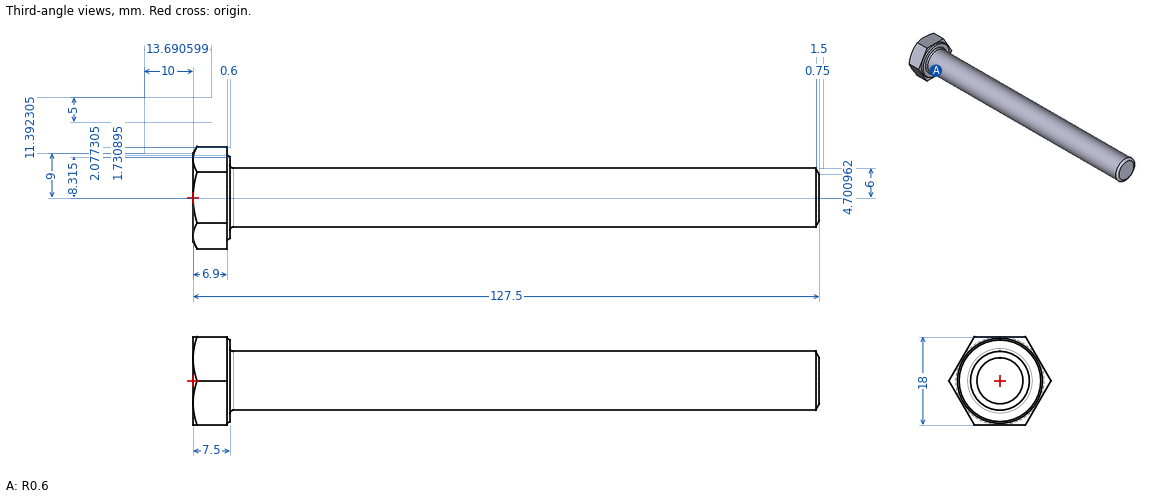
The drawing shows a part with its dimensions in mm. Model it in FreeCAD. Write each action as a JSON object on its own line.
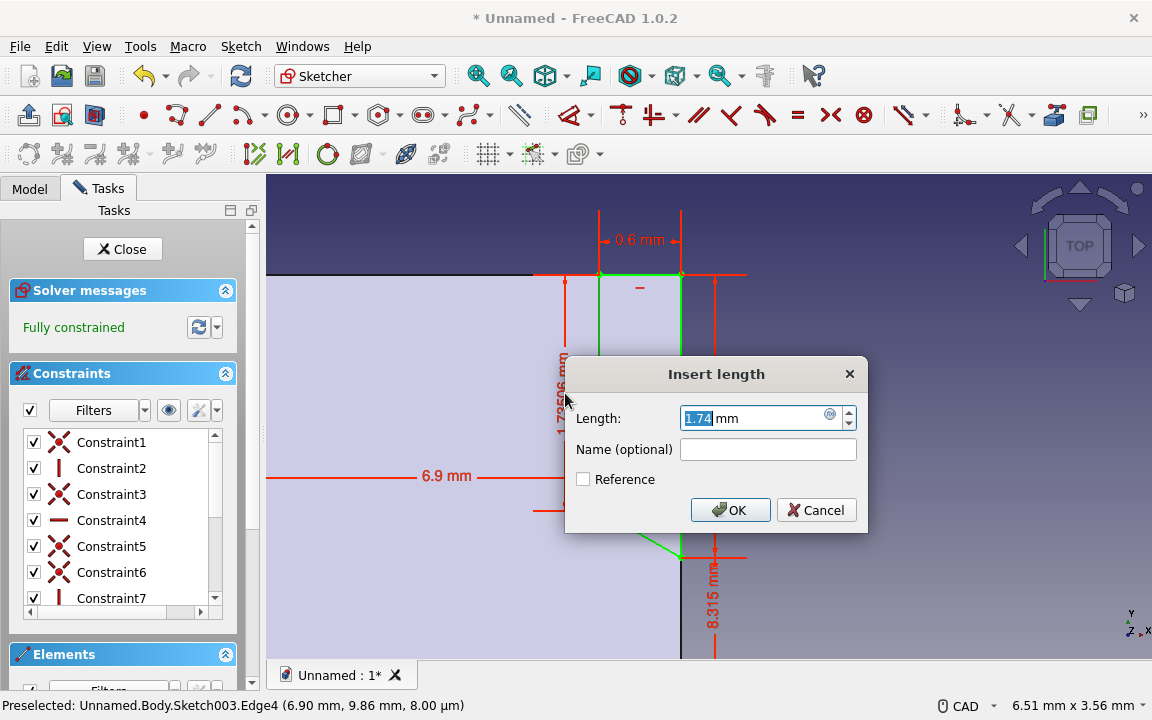
{"action": "type", "text": "1.730895"}
{"action": "key", "text": "Return"}
{"action": "key", "text": "Escape"}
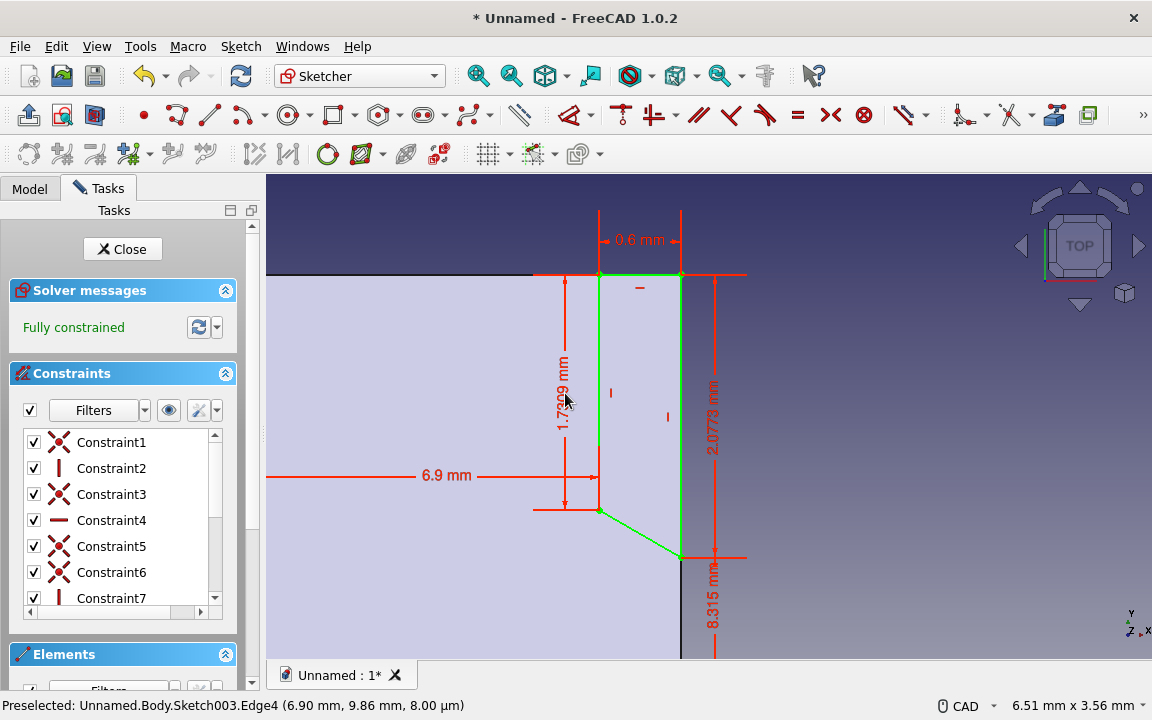
{"action": "left_click", "coordinate": [123, 249]}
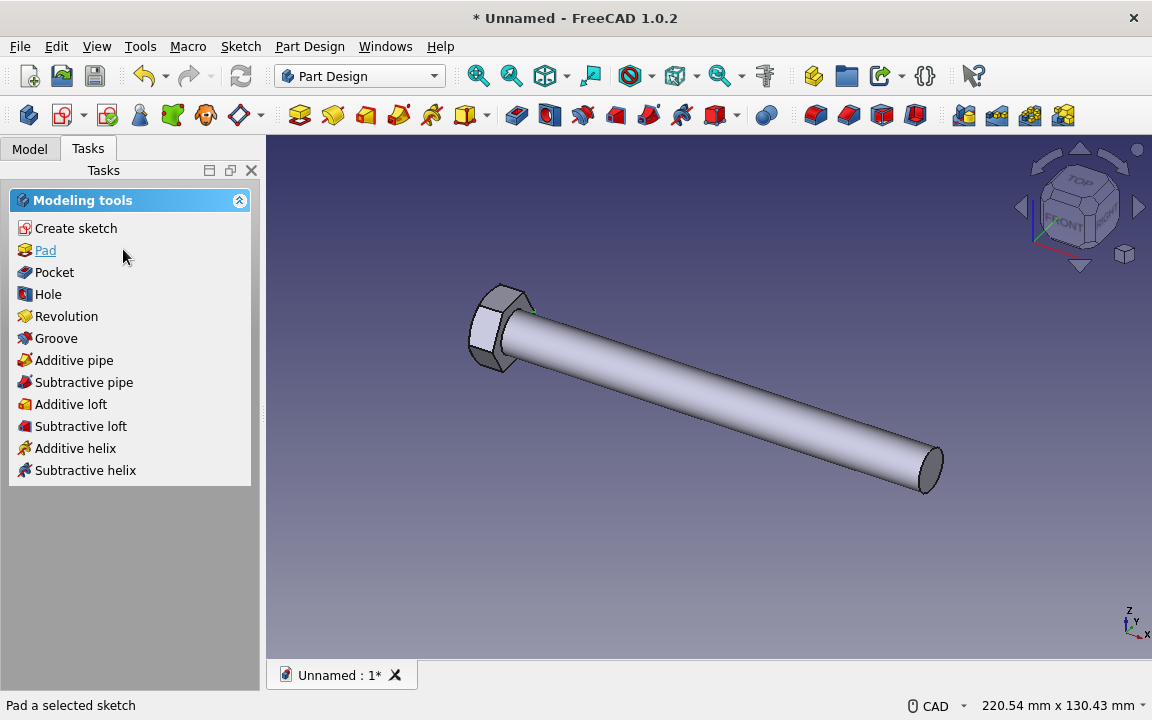
{"action": "left_click", "coordinate": [583, 116]}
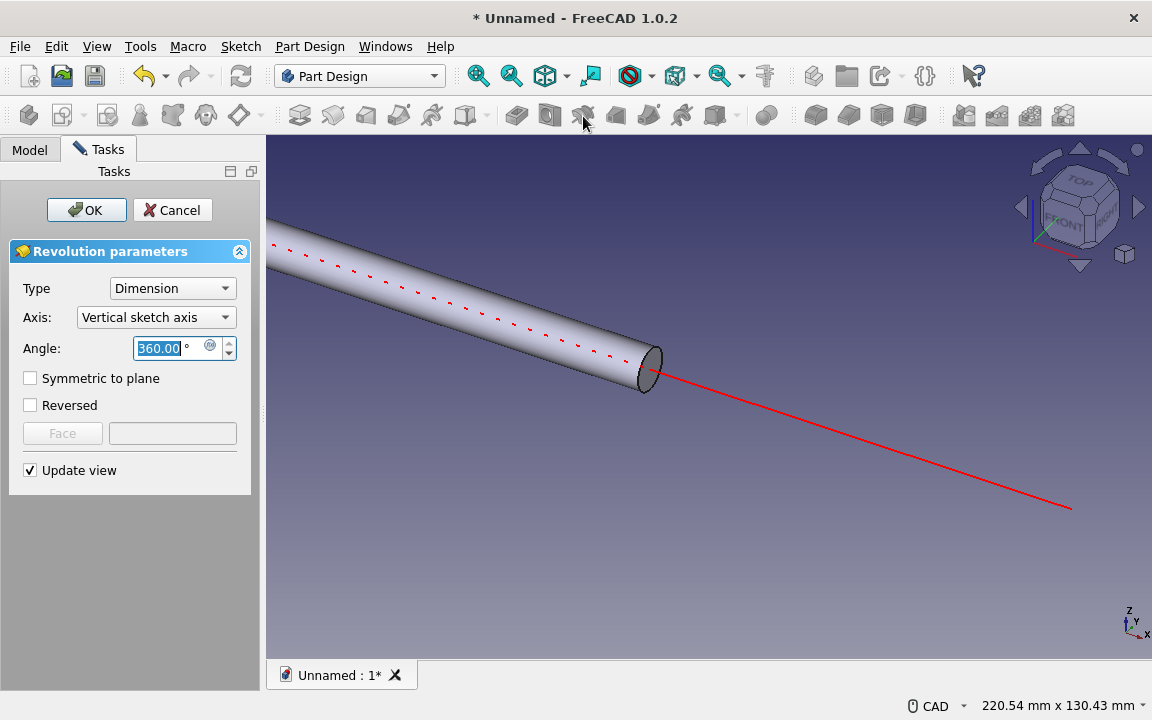
{"action": "left_click", "coordinate": [157, 318]}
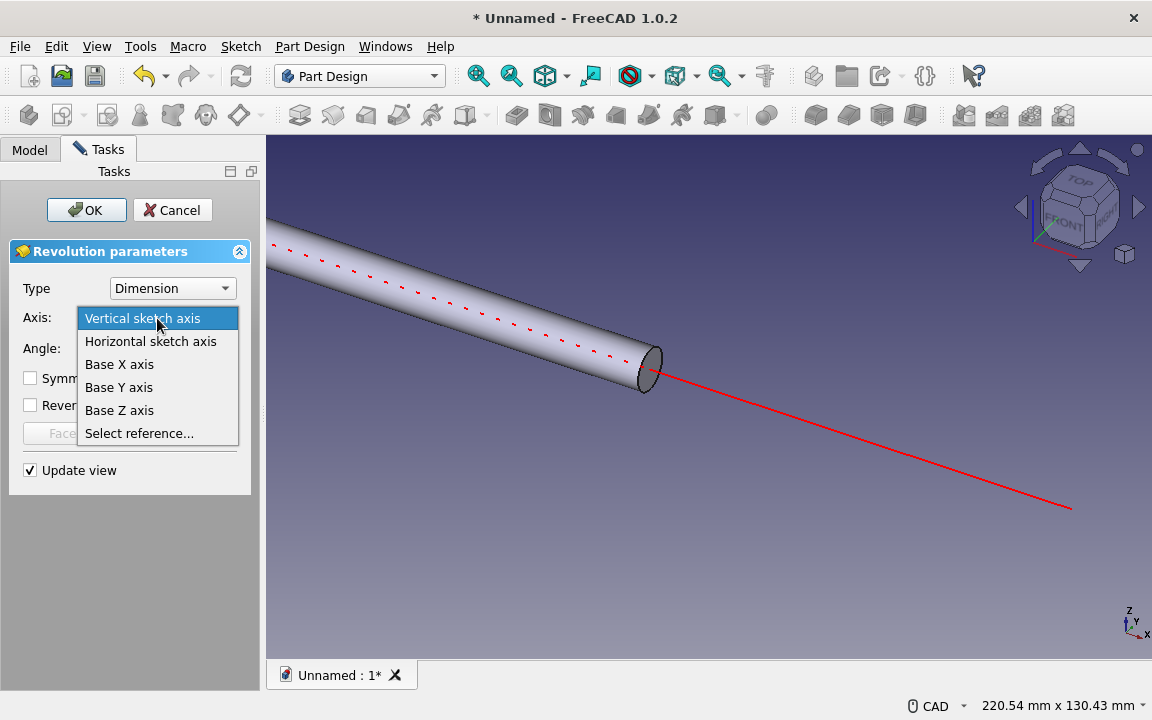
{"action": "left_click", "coordinate": [156, 342]}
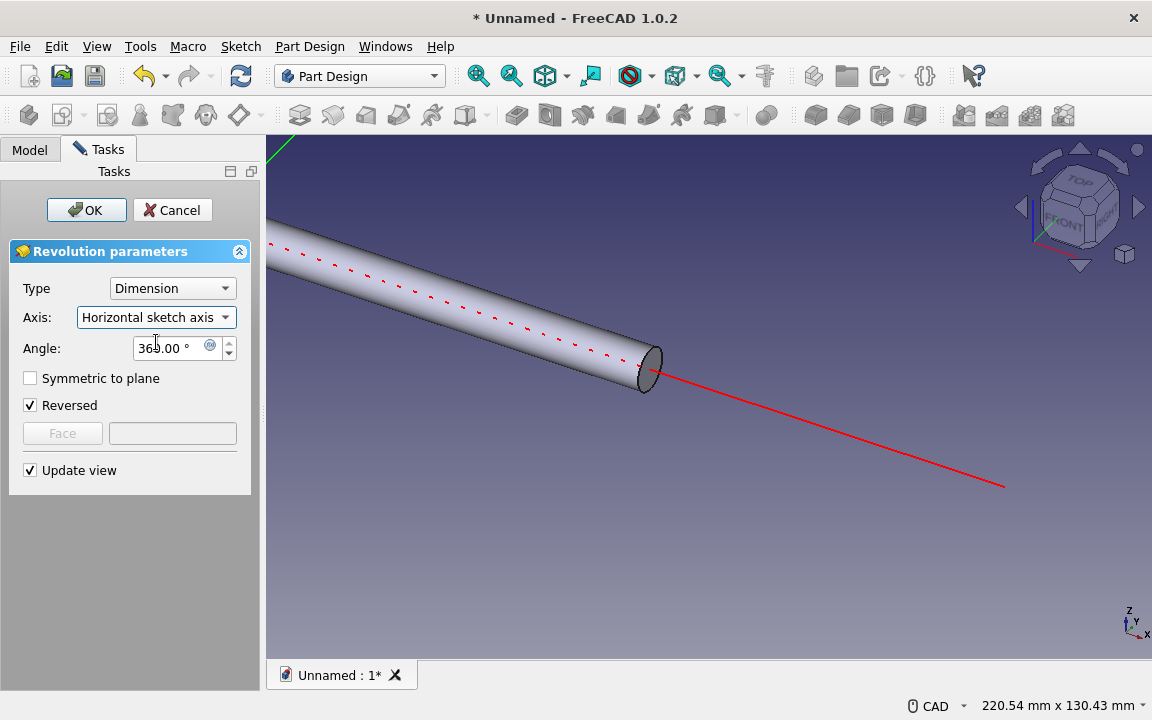
{"action": "left_click", "coordinate": [87, 210]}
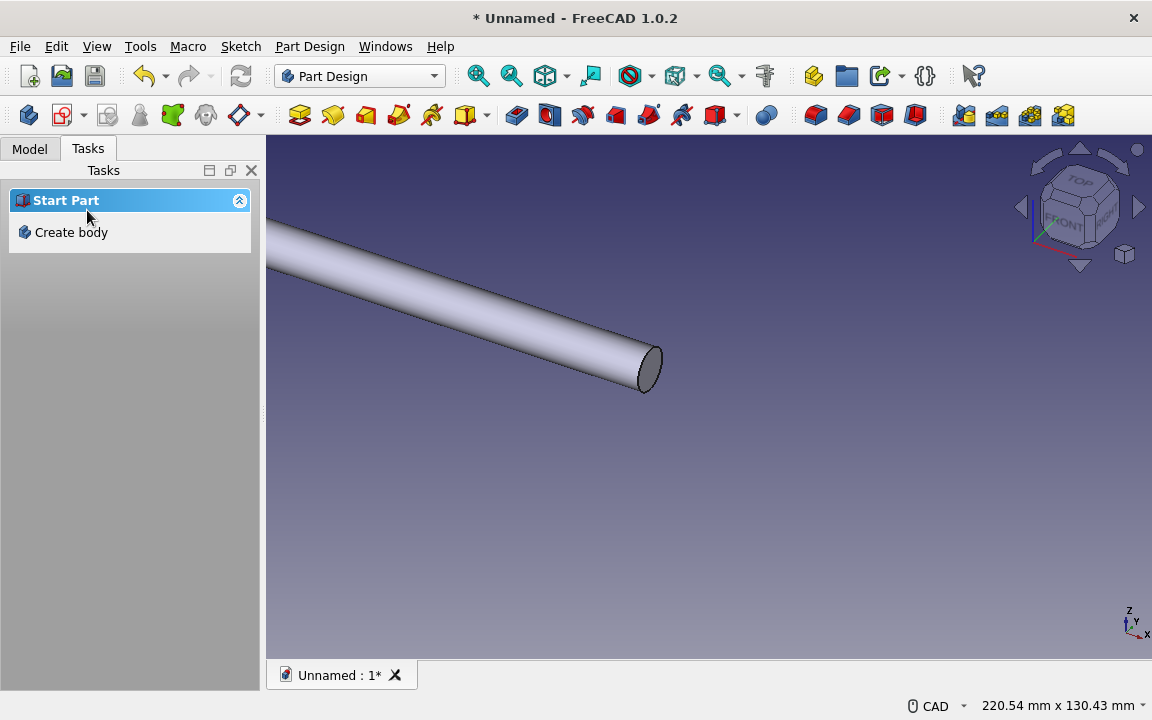
{"action": "left_click", "coordinate": [479, 76]}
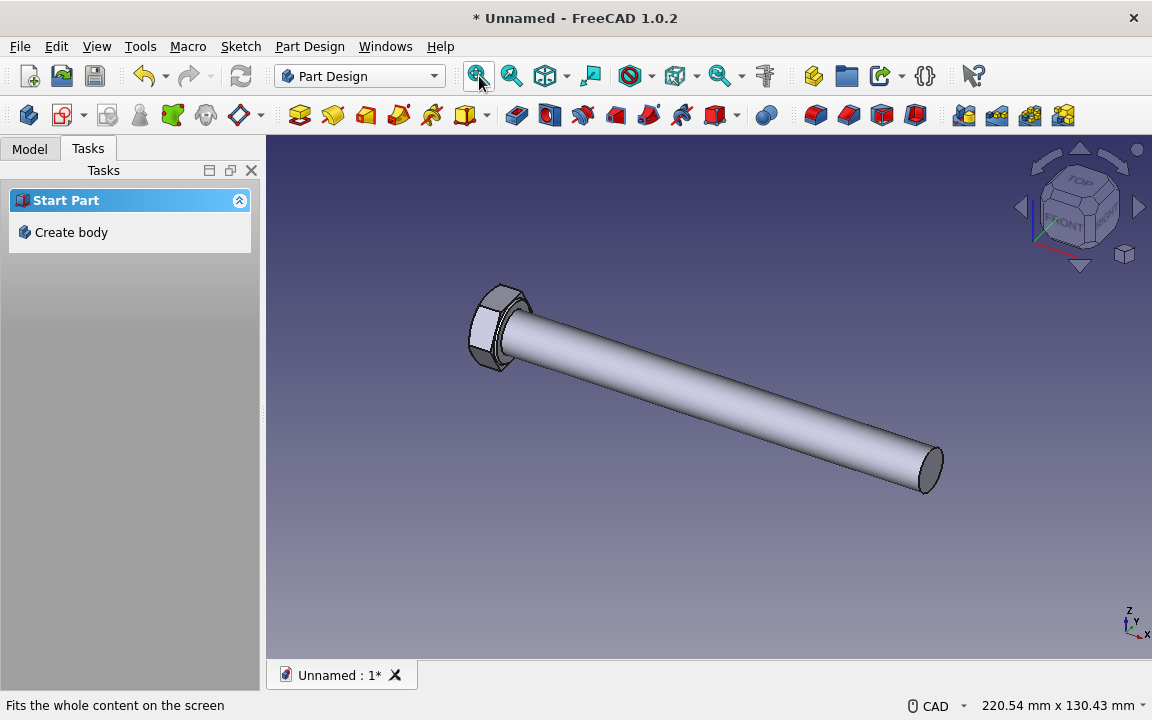
{"action": "key", "text": "0"}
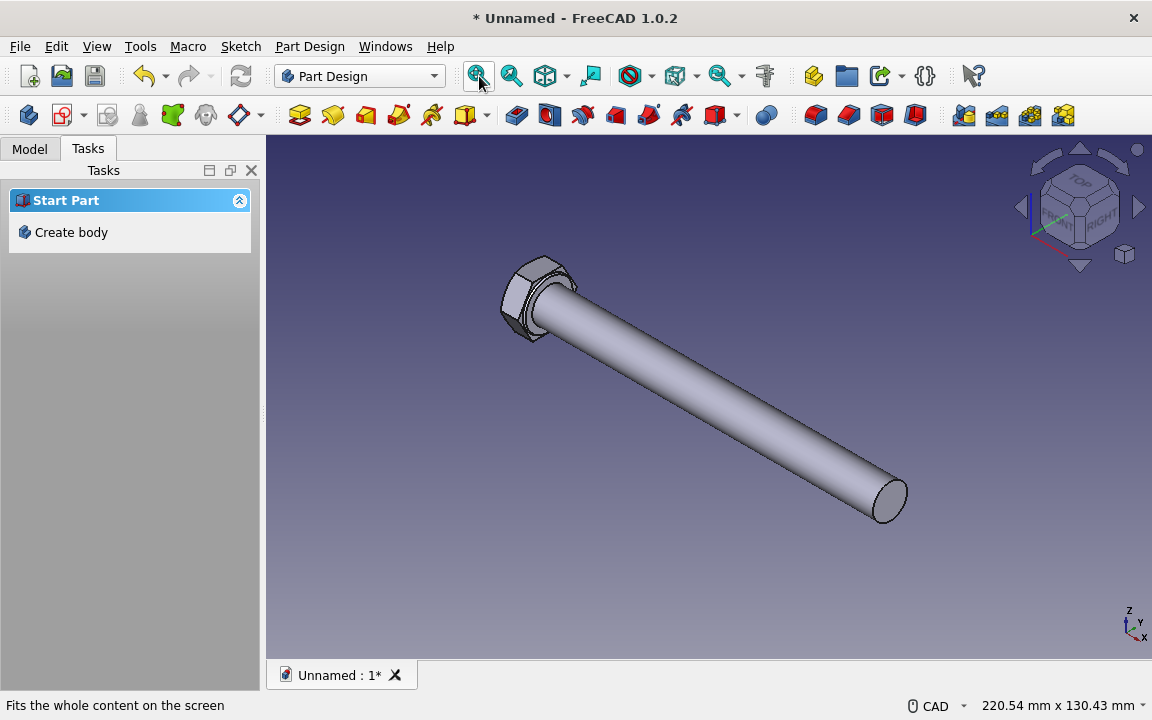
{"action": "key", "text": "2"}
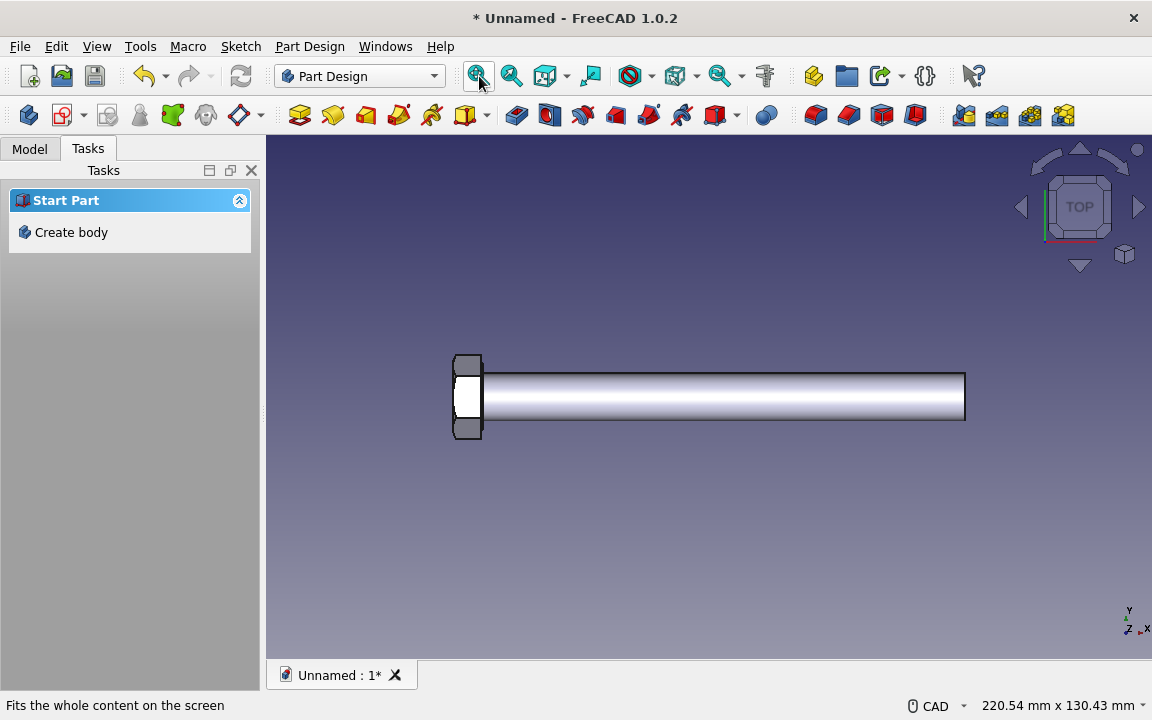
{"action": "key", "text": "1"}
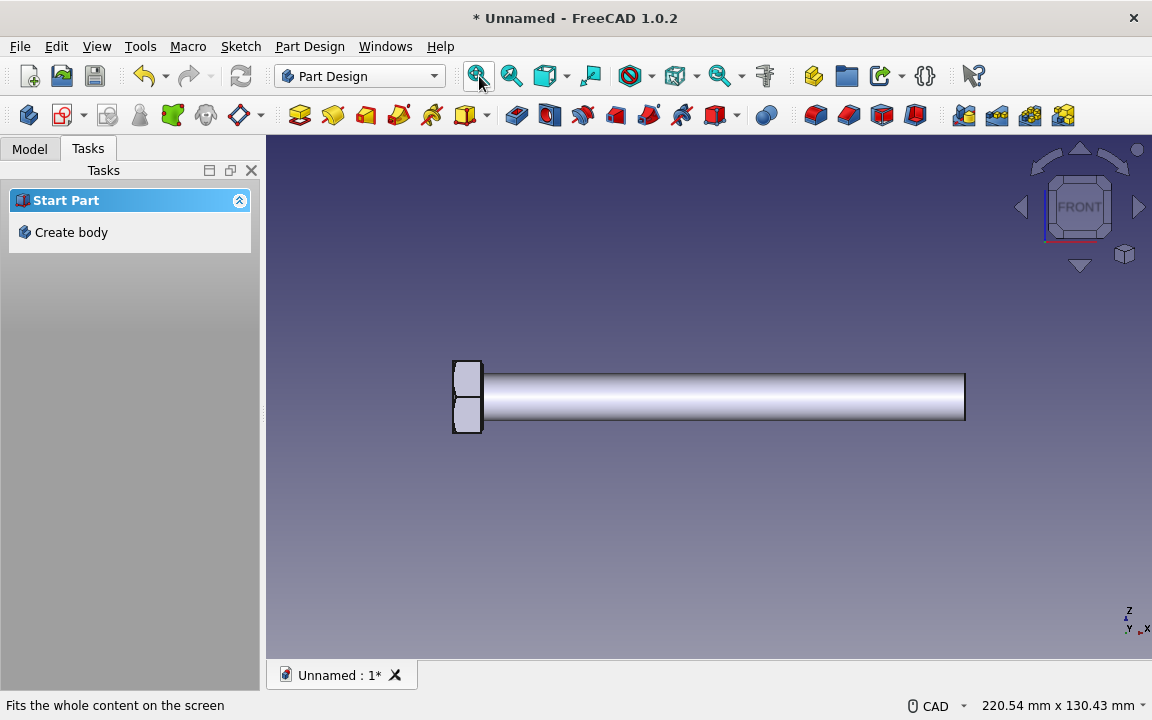
{"action": "key", "text": "3"}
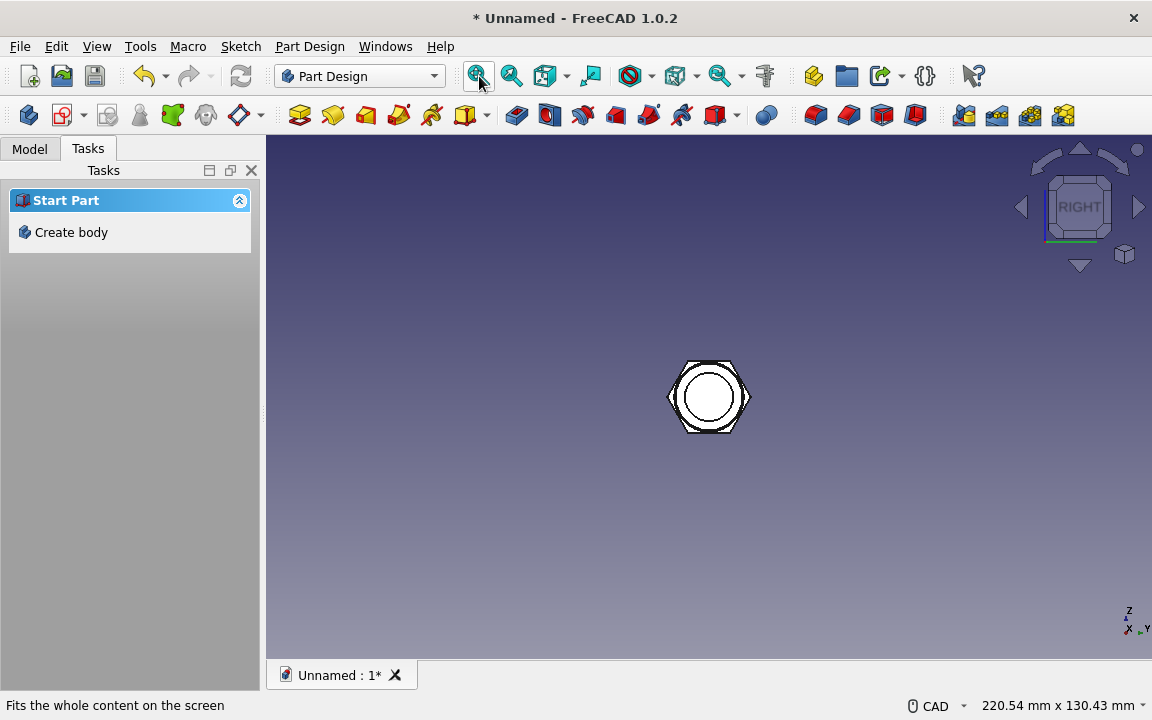
{"action": "left_click", "coordinate": [479, 76]}